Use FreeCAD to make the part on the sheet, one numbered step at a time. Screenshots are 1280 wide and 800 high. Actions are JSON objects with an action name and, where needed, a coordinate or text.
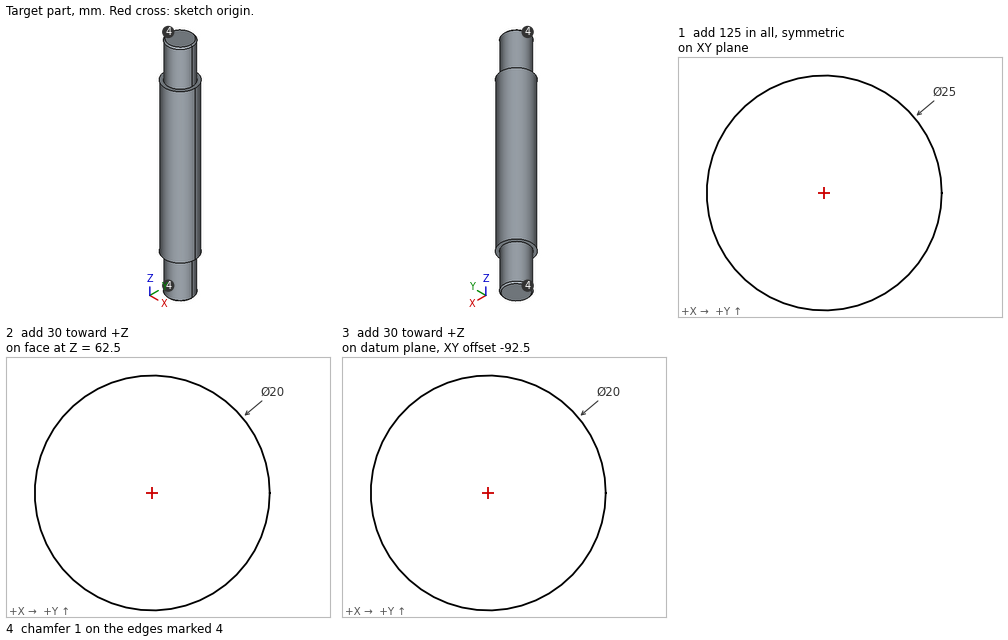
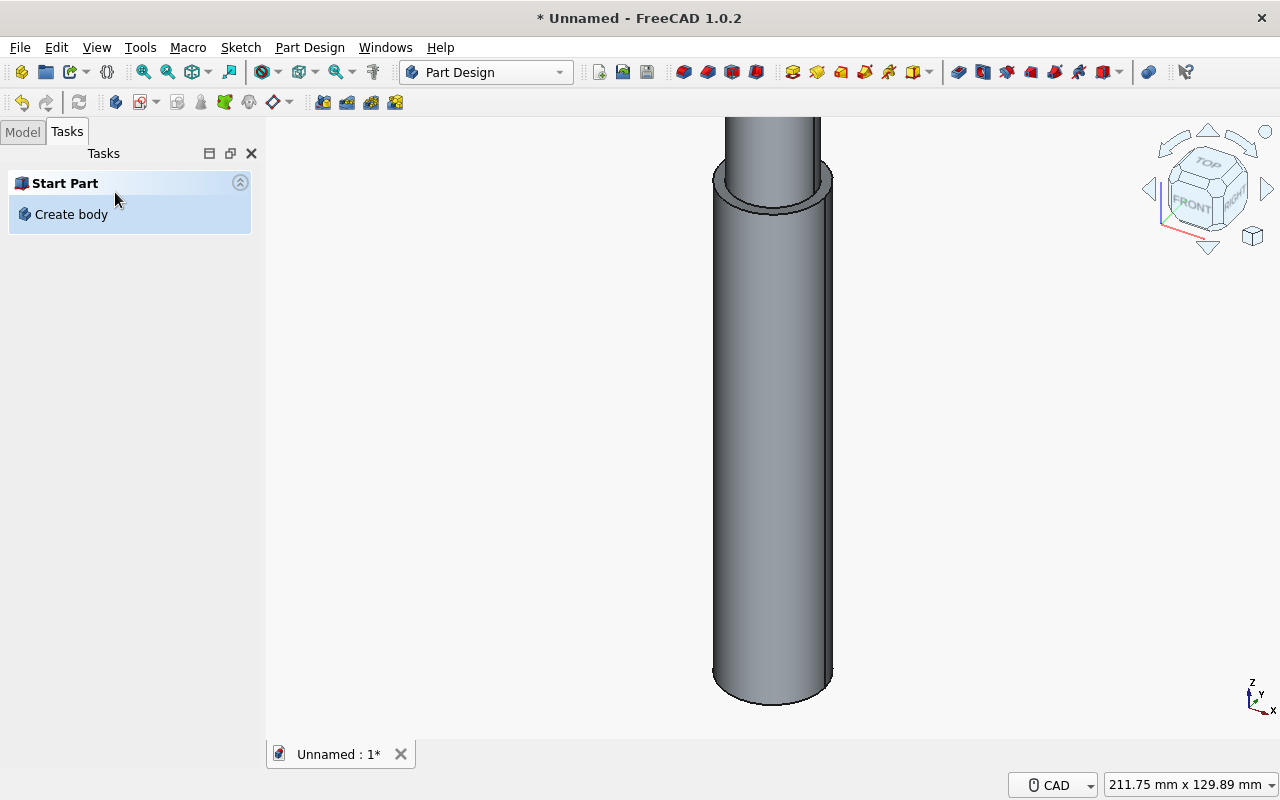
{"action": "left_click", "coordinate": [144, 72]}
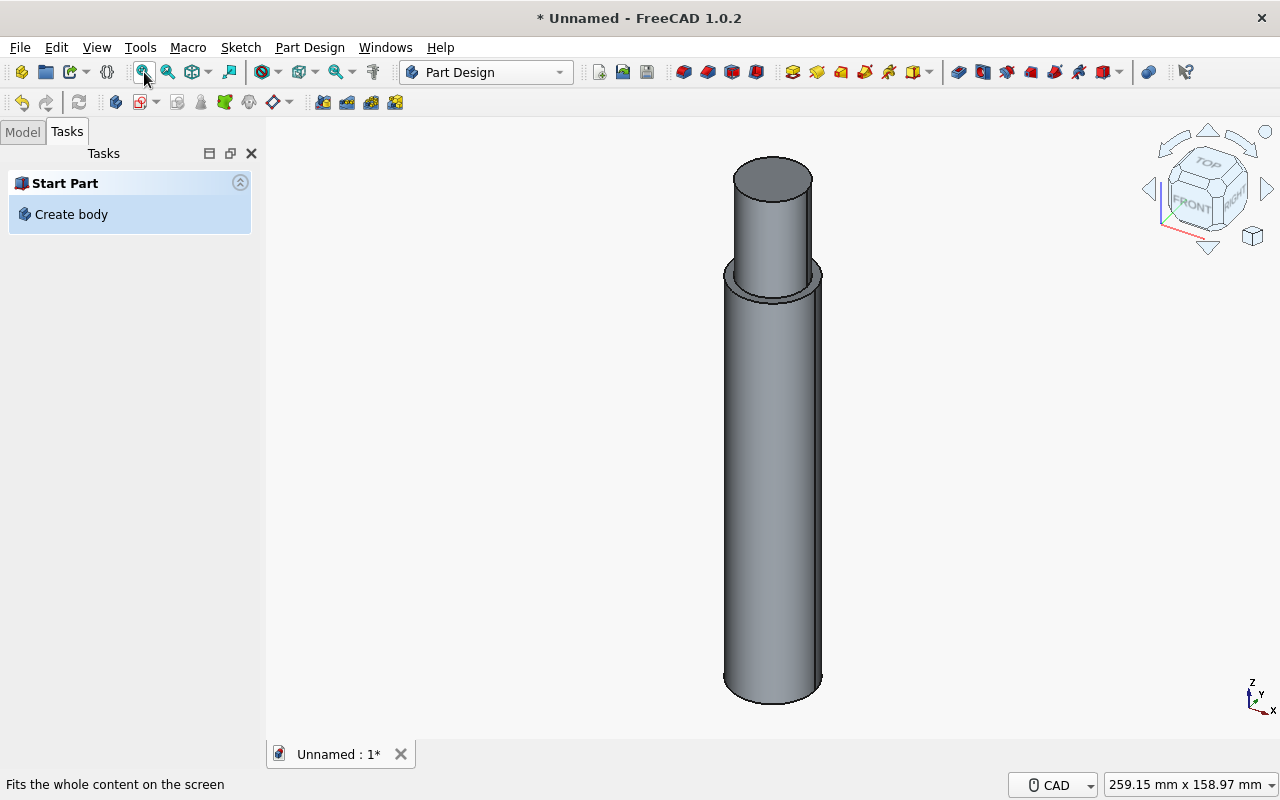
{"action": "left_click", "coordinate": [23, 131]}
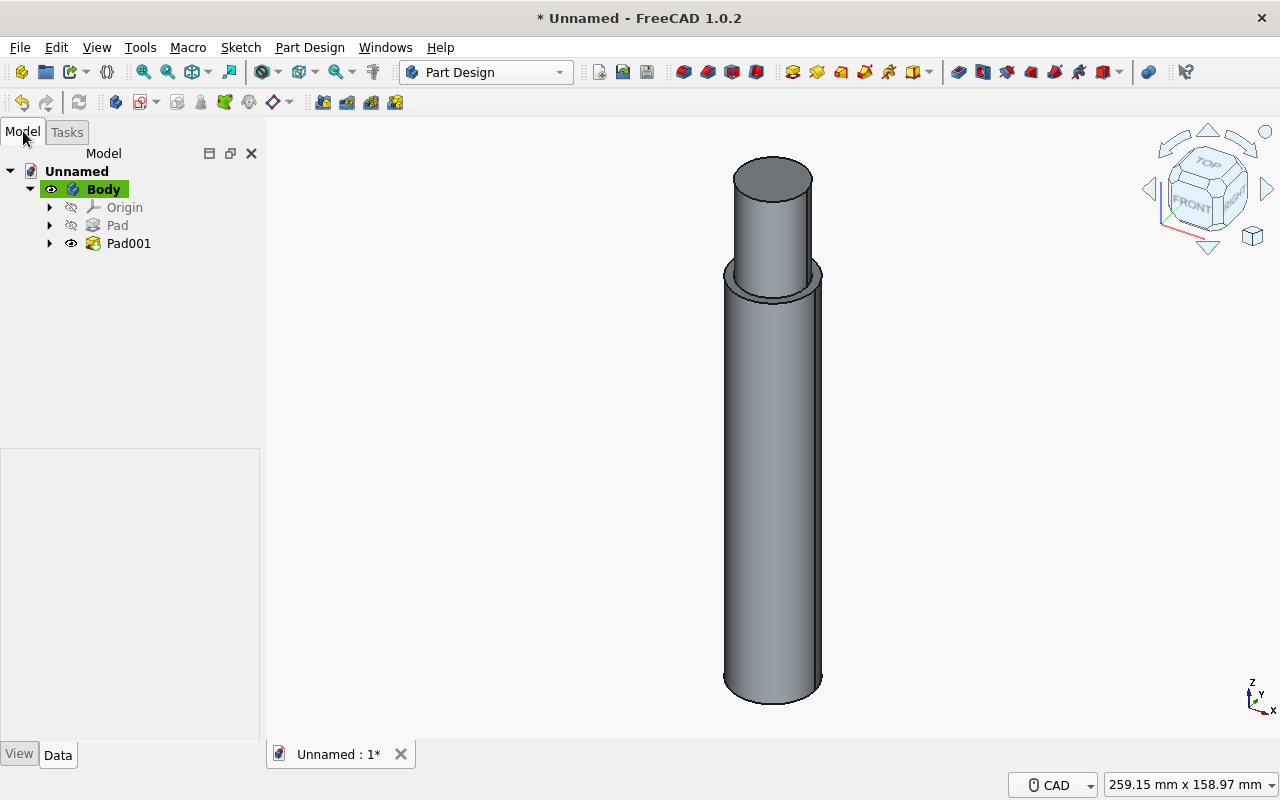
{"action": "left_click", "coordinate": [50, 207]}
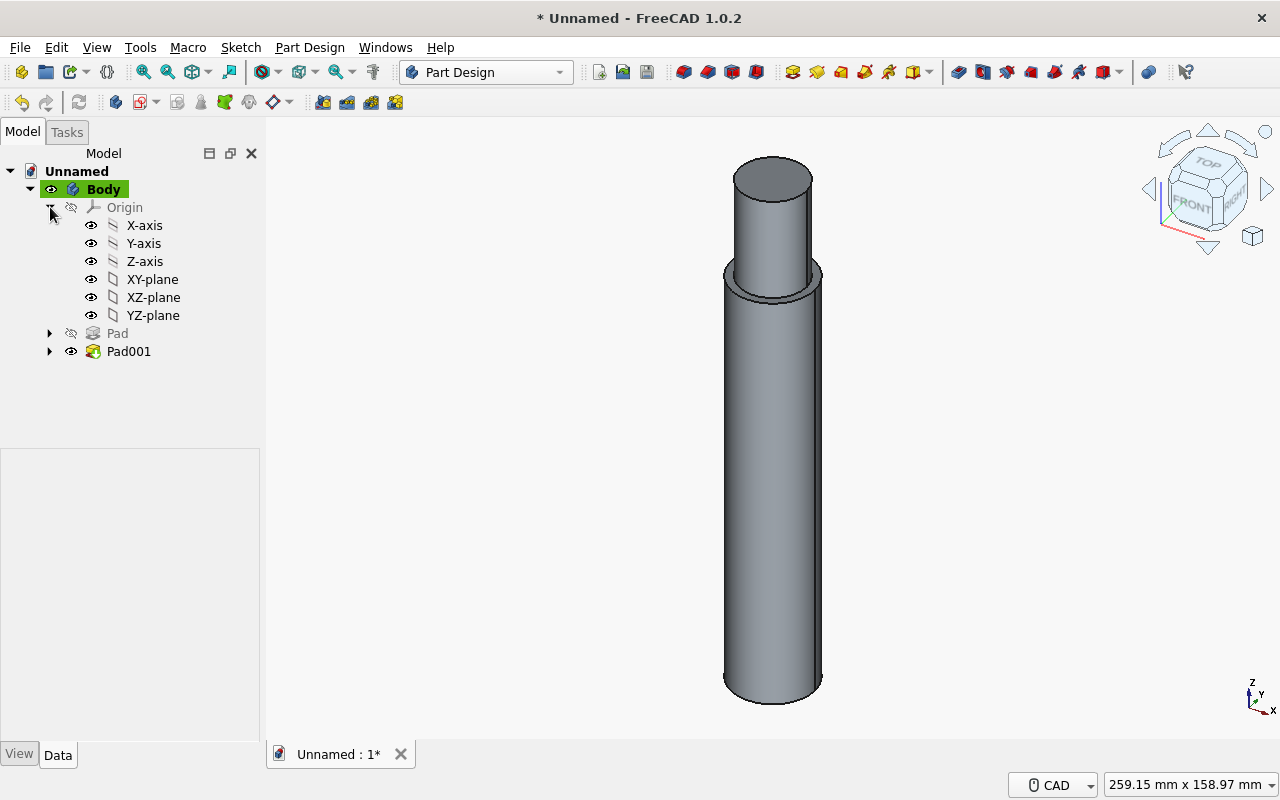
{"action": "left_click", "coordinate": [136, 279]}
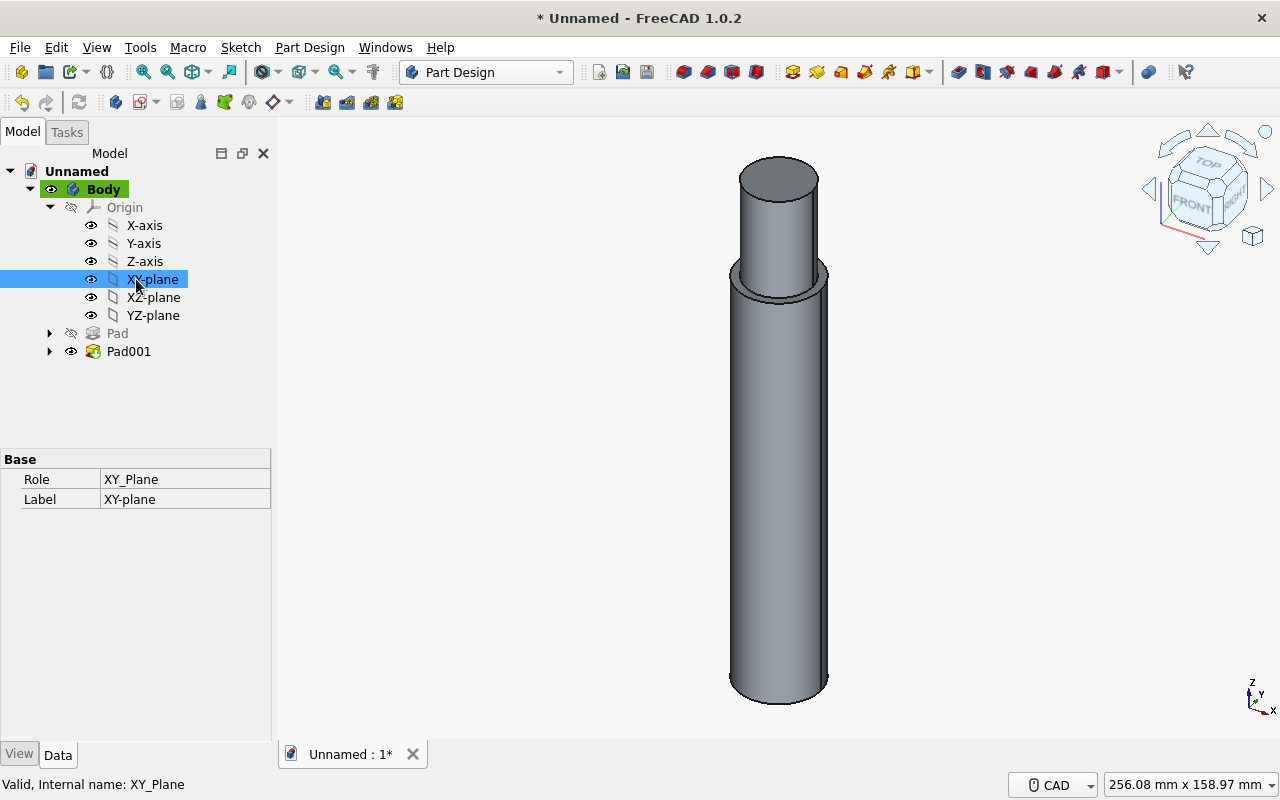
{"action": "left_click", "coordinate": [274, 102]}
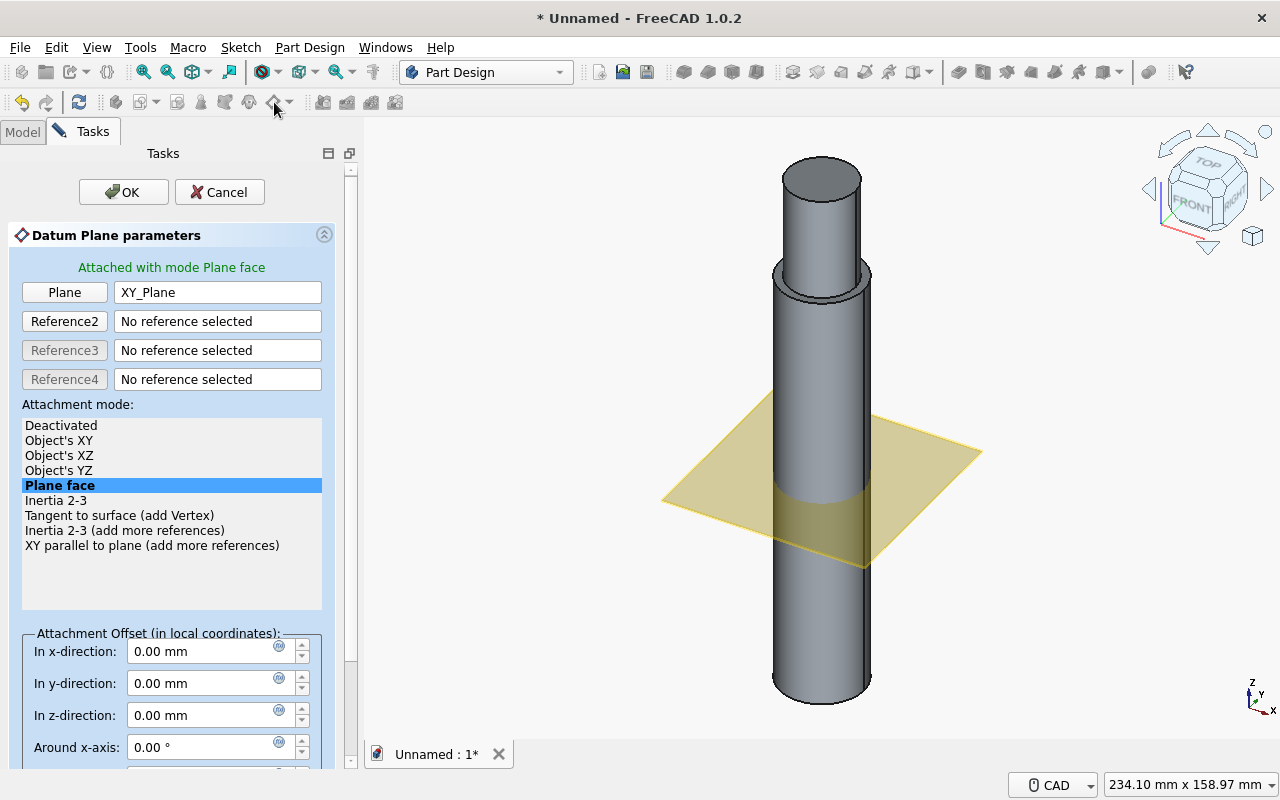
{"action": "triple_click", "coordinate": [210, 715]}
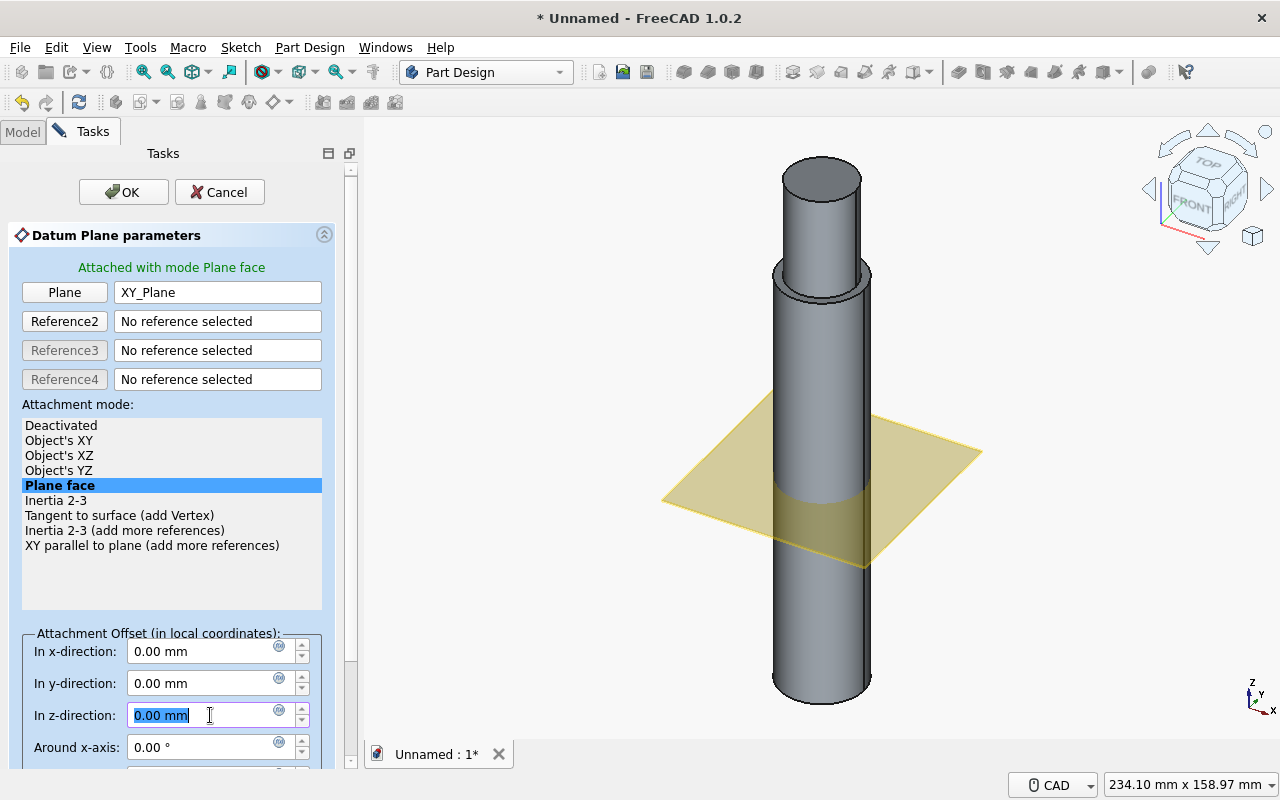
{"action": "type", "text": "-92.5"}
{"action": "key", "text": "Tab"}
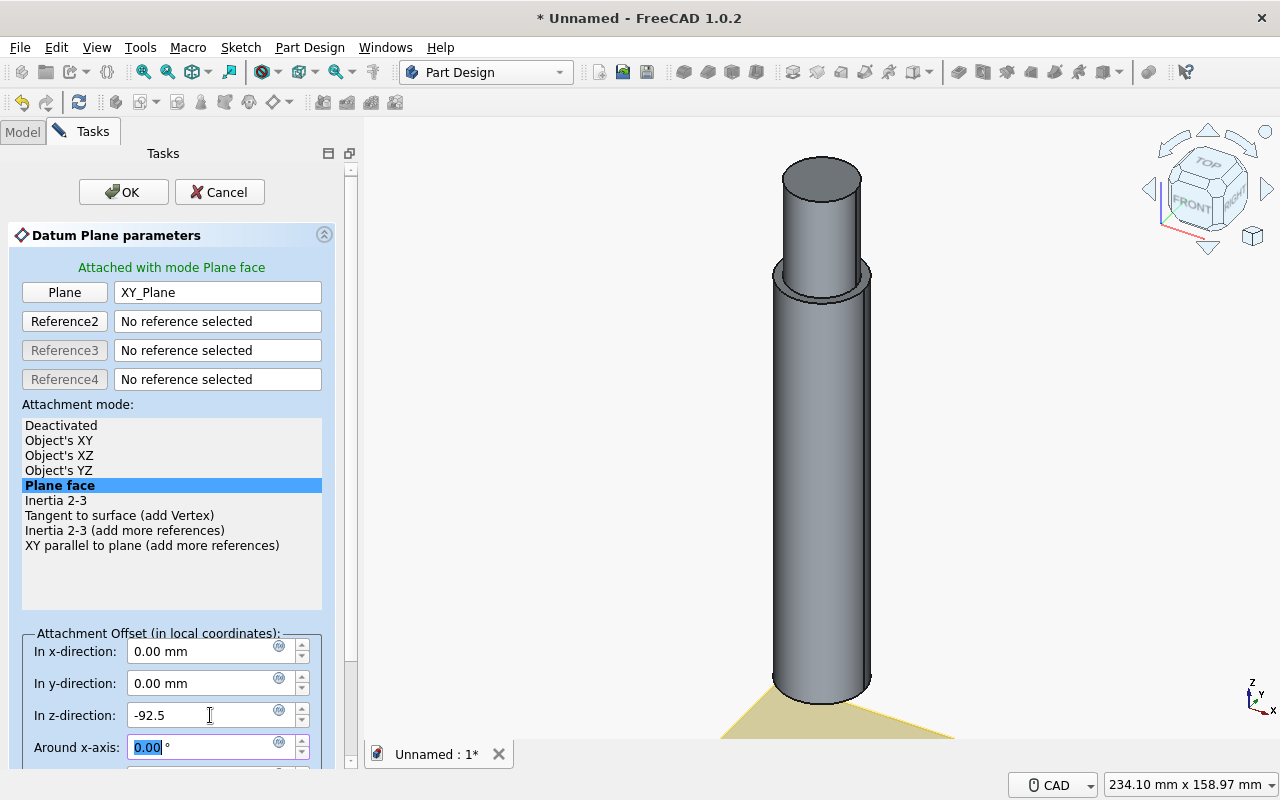
{"action": "left_click", "coordinate": [124, 192]}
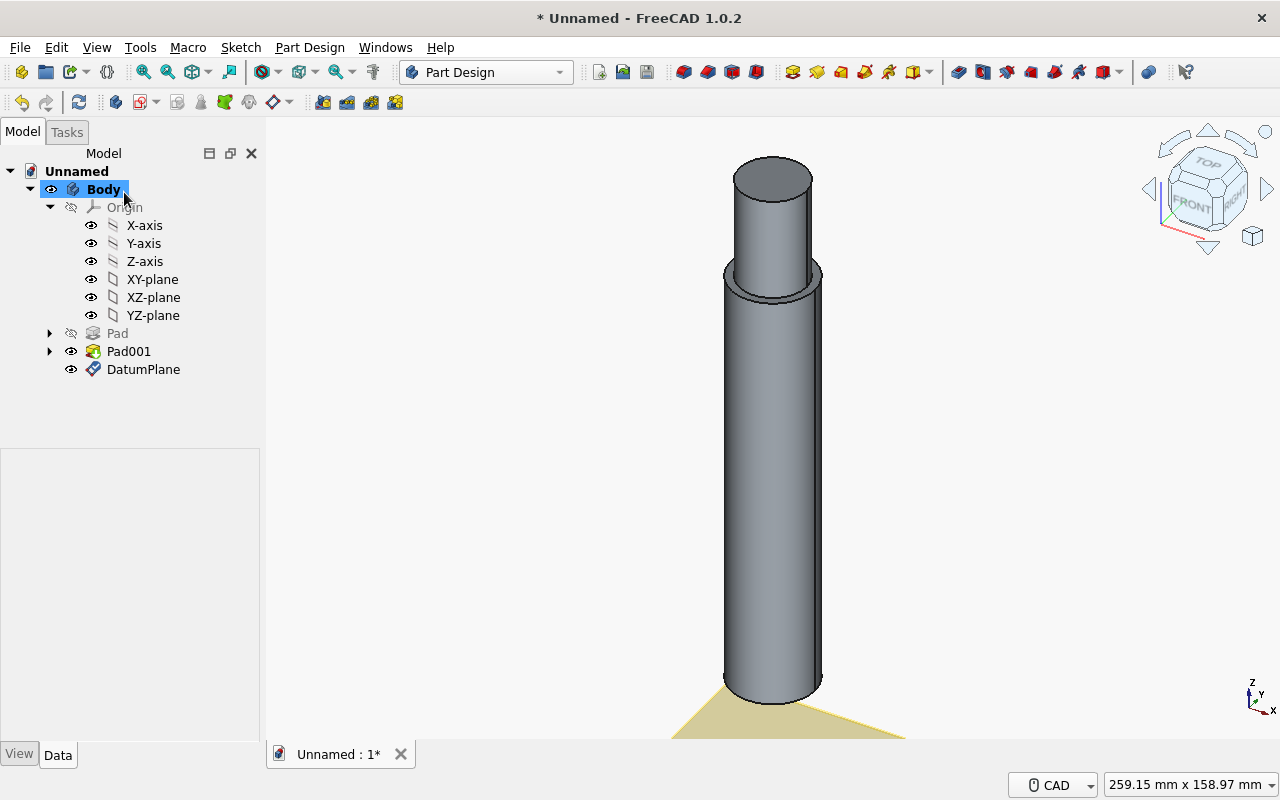
{"action": "left_click", "coordinate": [116, 369]}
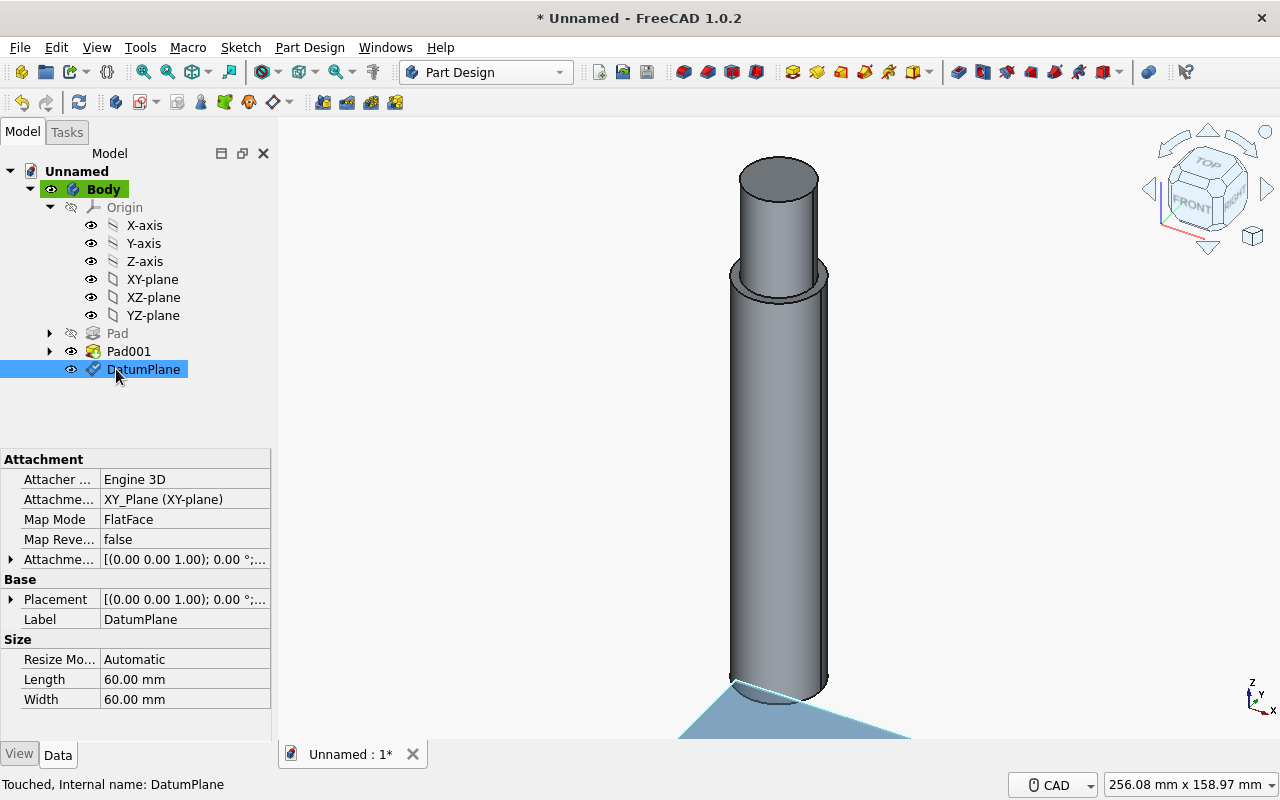
{"action": "left_click", "coordinate": [140, 102]}